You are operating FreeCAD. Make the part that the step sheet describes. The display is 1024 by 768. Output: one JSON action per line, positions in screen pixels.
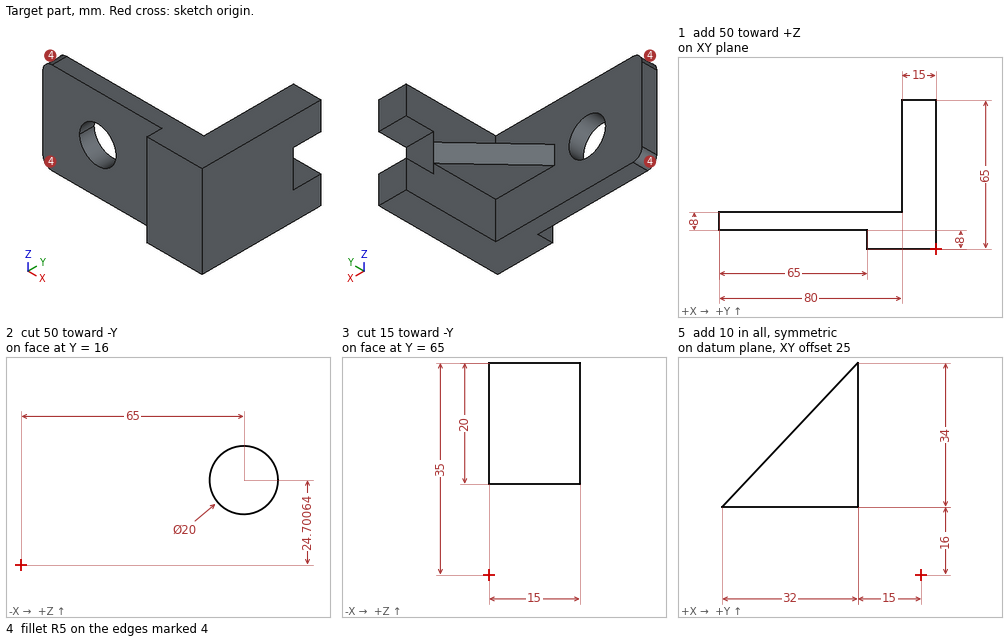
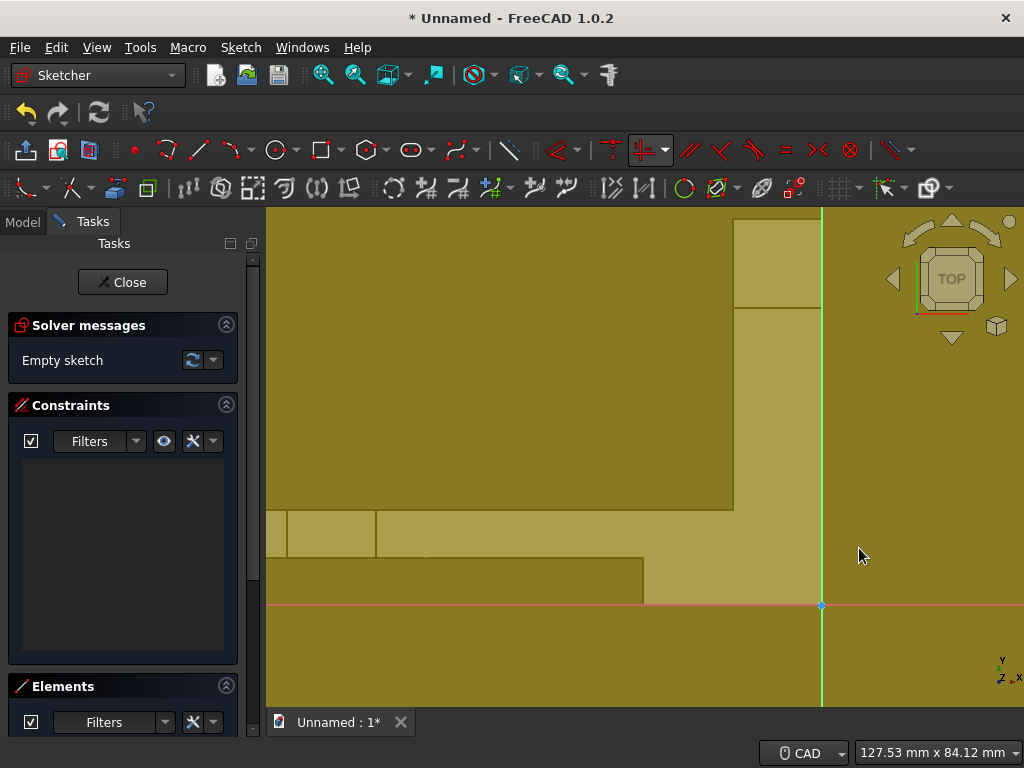
{"action": "left_click", "coordinate": [168, 150]}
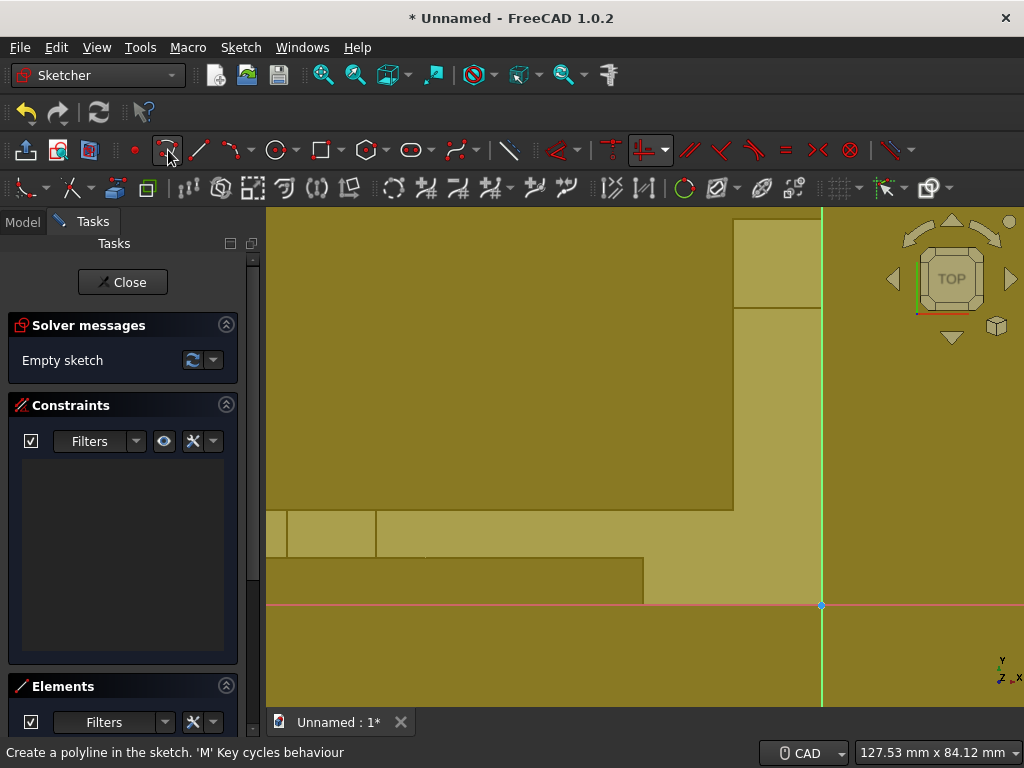
{"action": "left_click", "coordinate": [733, 510]}
{"action": "left_click", "coordinate": [542, 510]}
{"action": "left_click", "coordinate": [733, 308]}
{"action": "left_click", "coordinate": [733, 511]}
{"action": "key", "text": "Escape"}
{"action": "key", "text": "Escape"}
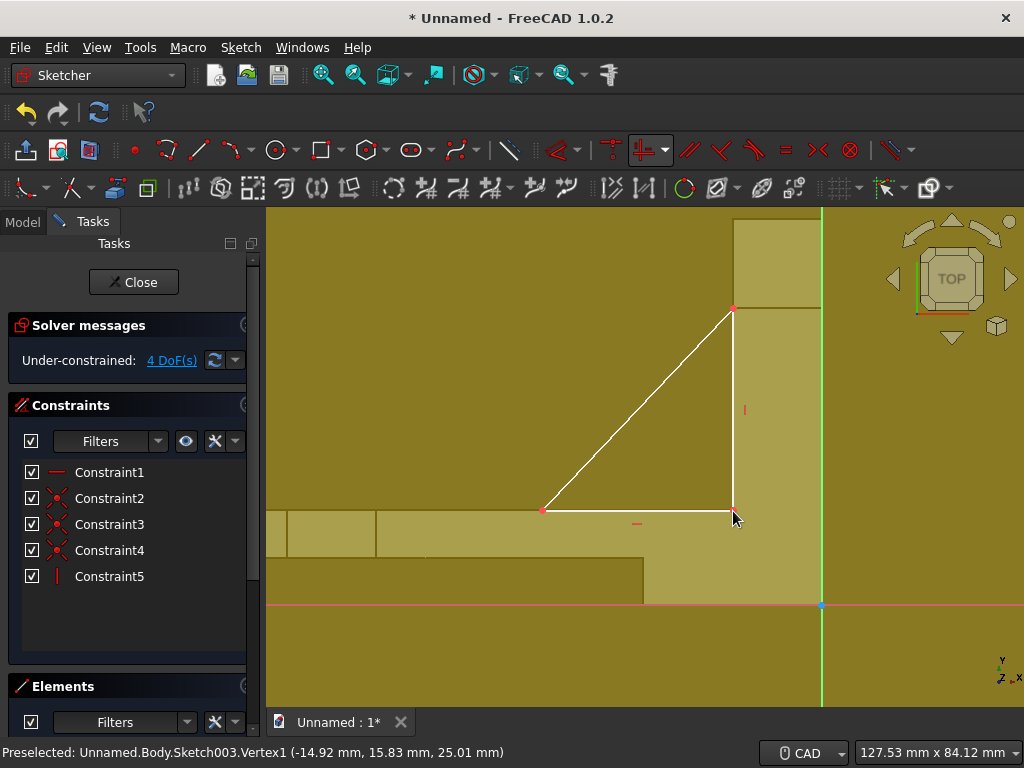
{"action": "key", "text": "d"}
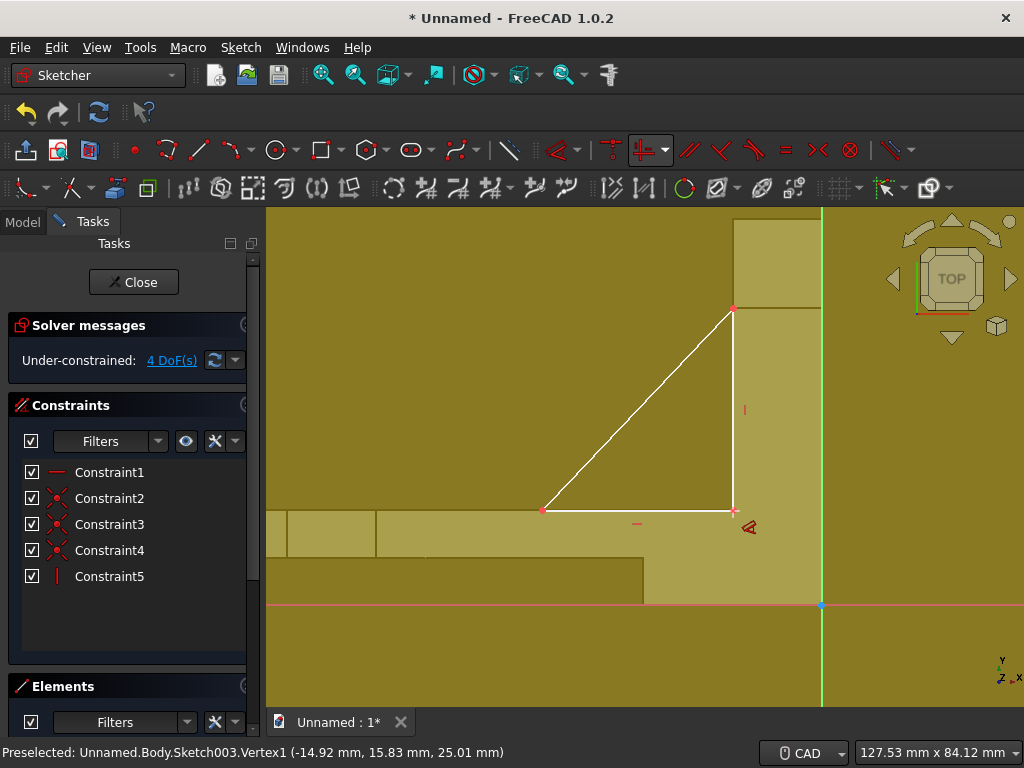
{"action": "left_click", "coordinate": [676, 511]}
{"action": "left_click", "coordinate": [637, 545]}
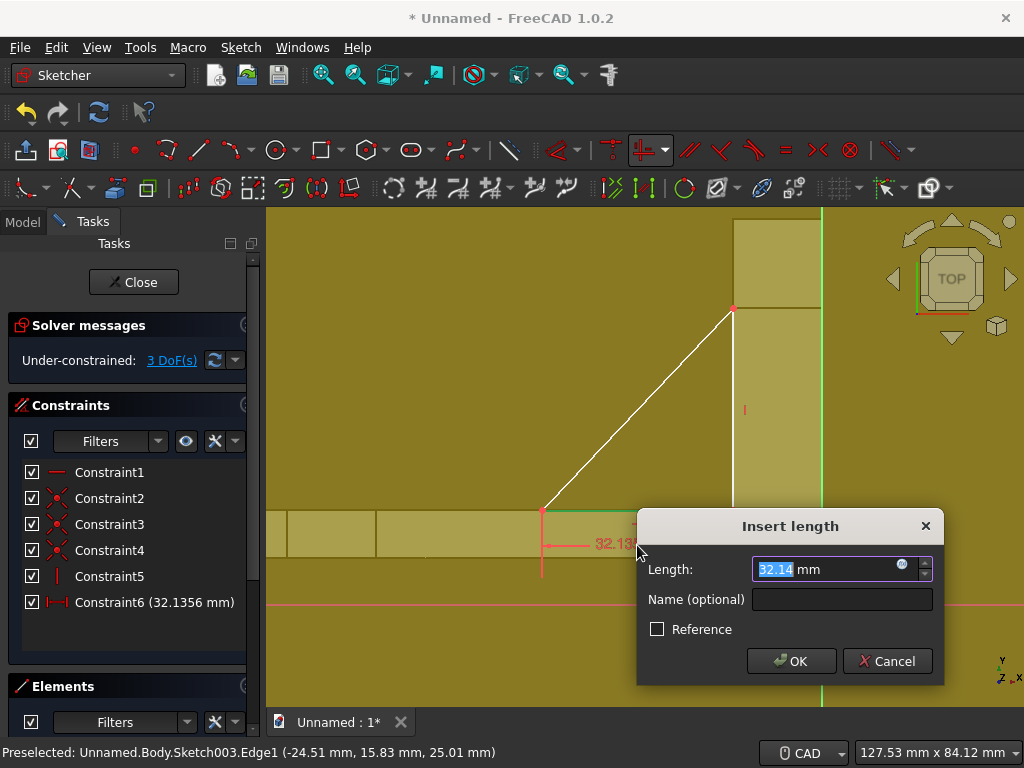
{"action": "type", "text": "32"}
{"action": "key", "text": "Return"}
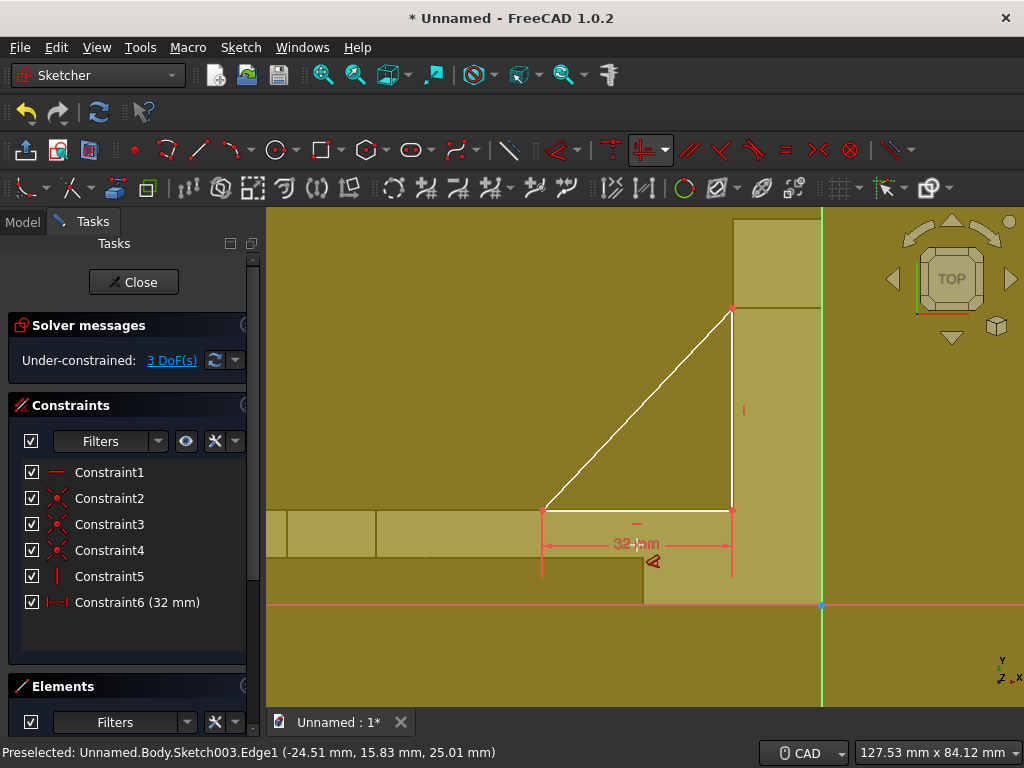
{"action": "left_click", "coordinate": [732, 370]}
{"action": "left_click", "coordinate": [766, 410]}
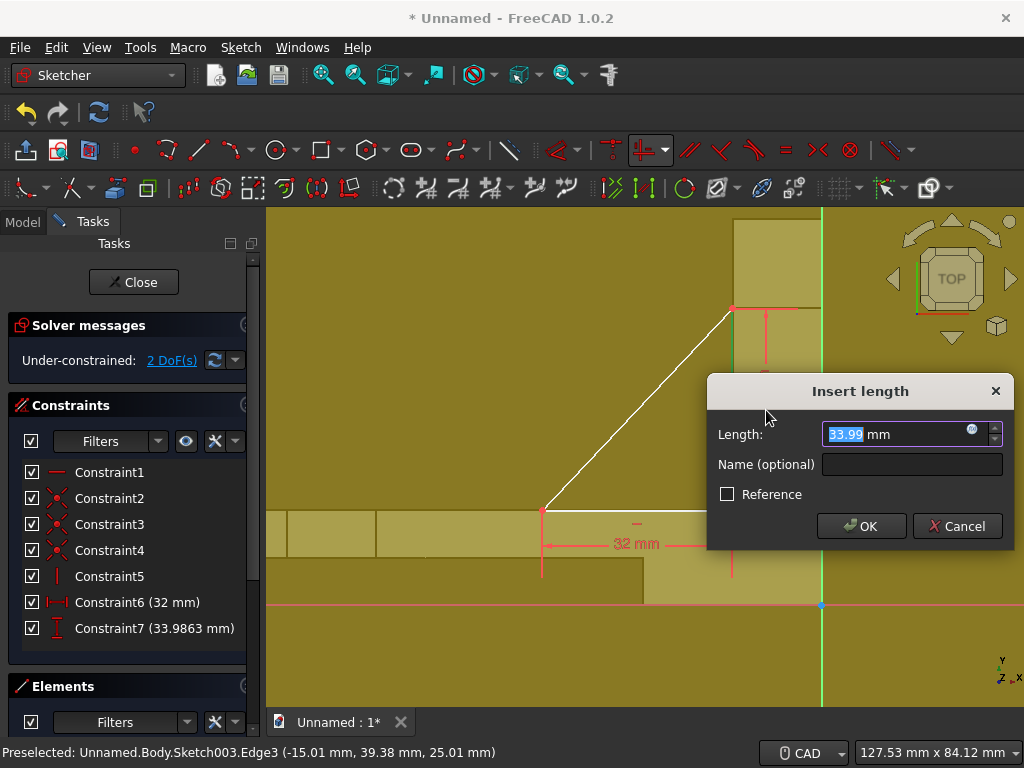
{"action": "type", "text": "34"}
{"action": "key", "text": "Return"}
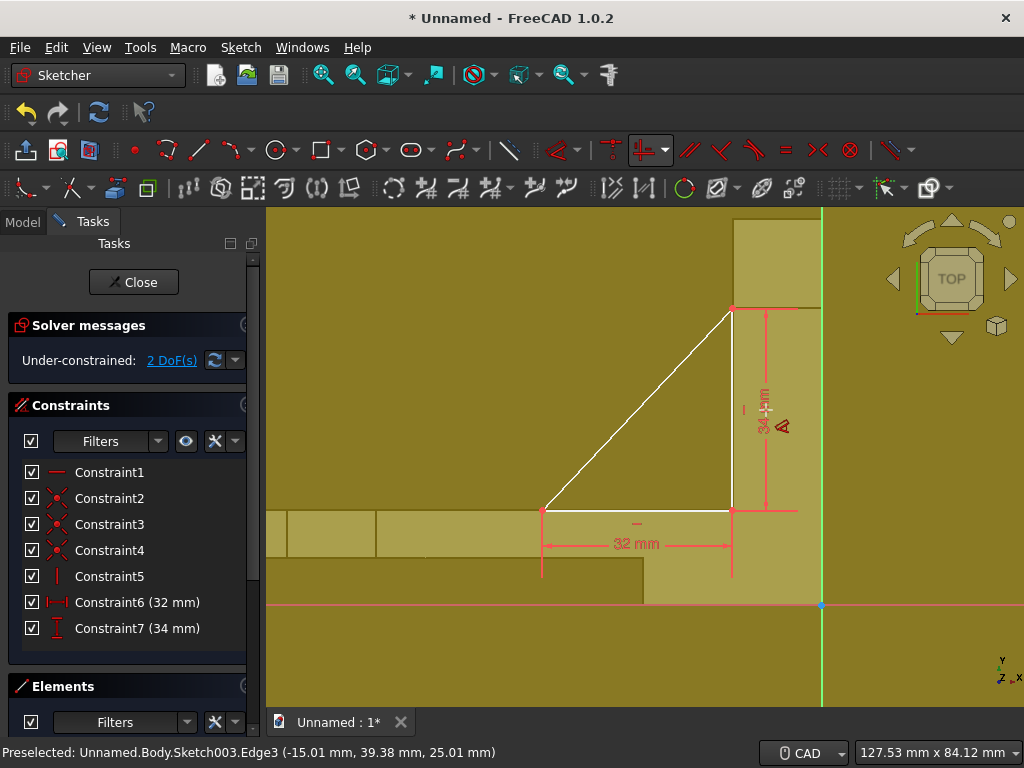
{"action": "left_click", "coordinate": [732, 511]}
{"action": "left_click", "coordinate": [777, 639]}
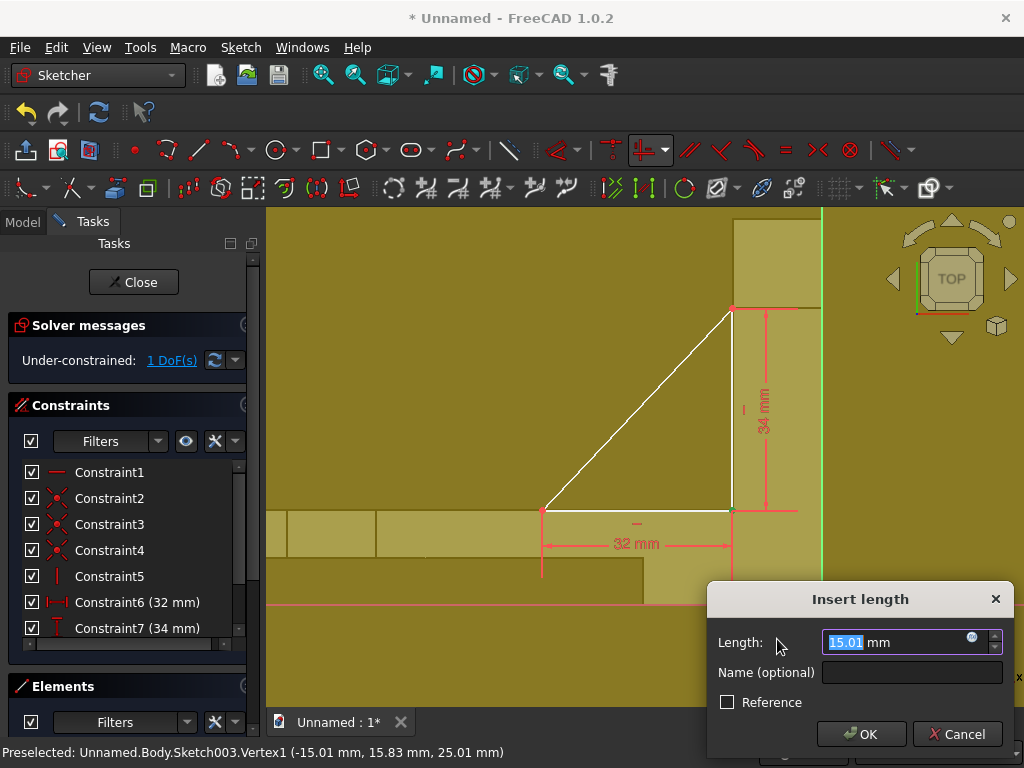
{"action": "type", "text": "15"}
{"action": "key", "text": "Return"}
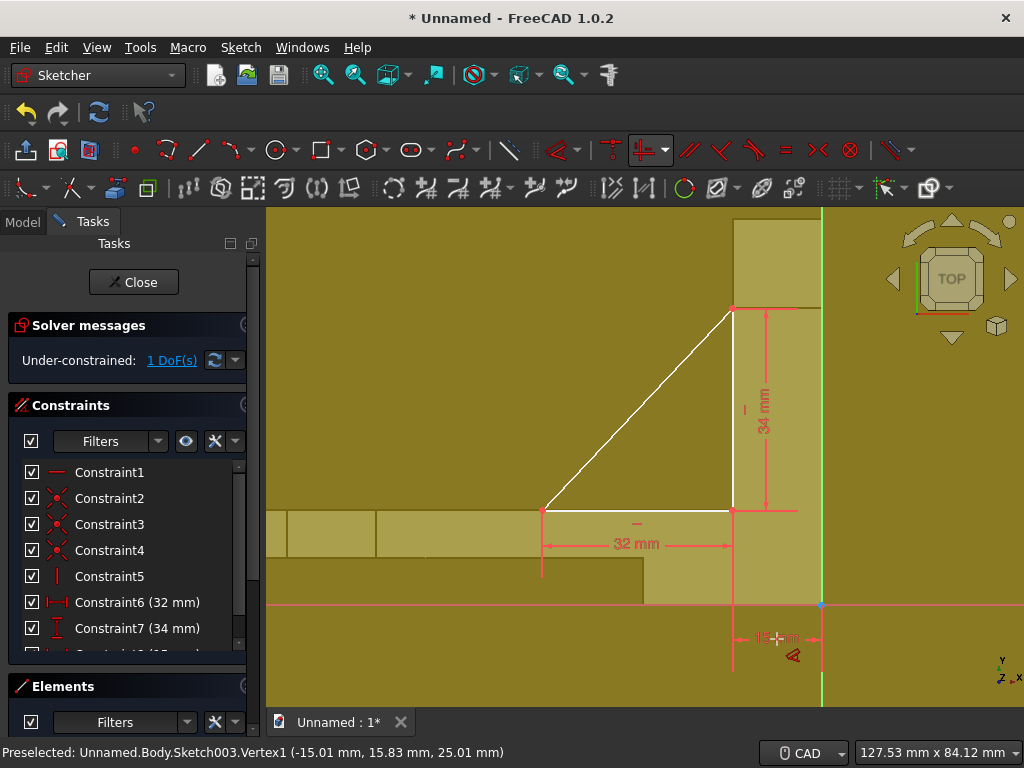
{"action": "left_click", "coordinate": [733, 511]}
{"action": "left_click", "coordinate": [856, 558]}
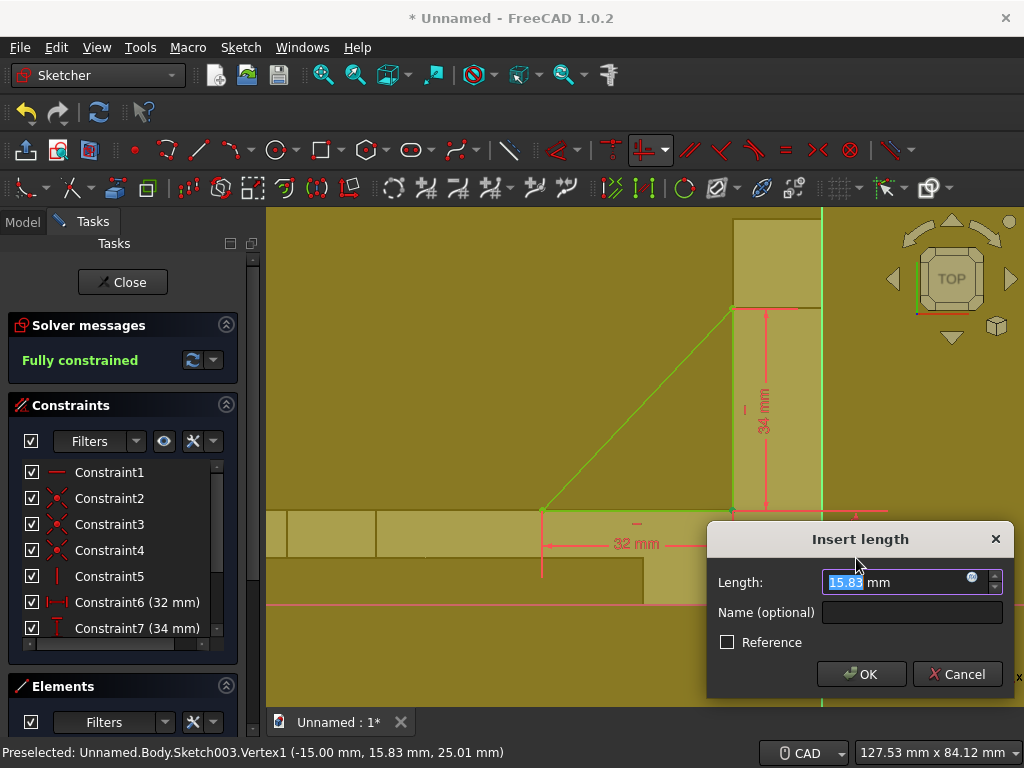
{"action": "type", "text": "16"}
{"action": "key", "text": "Return"}
{"action": "key", "text": "Escape"}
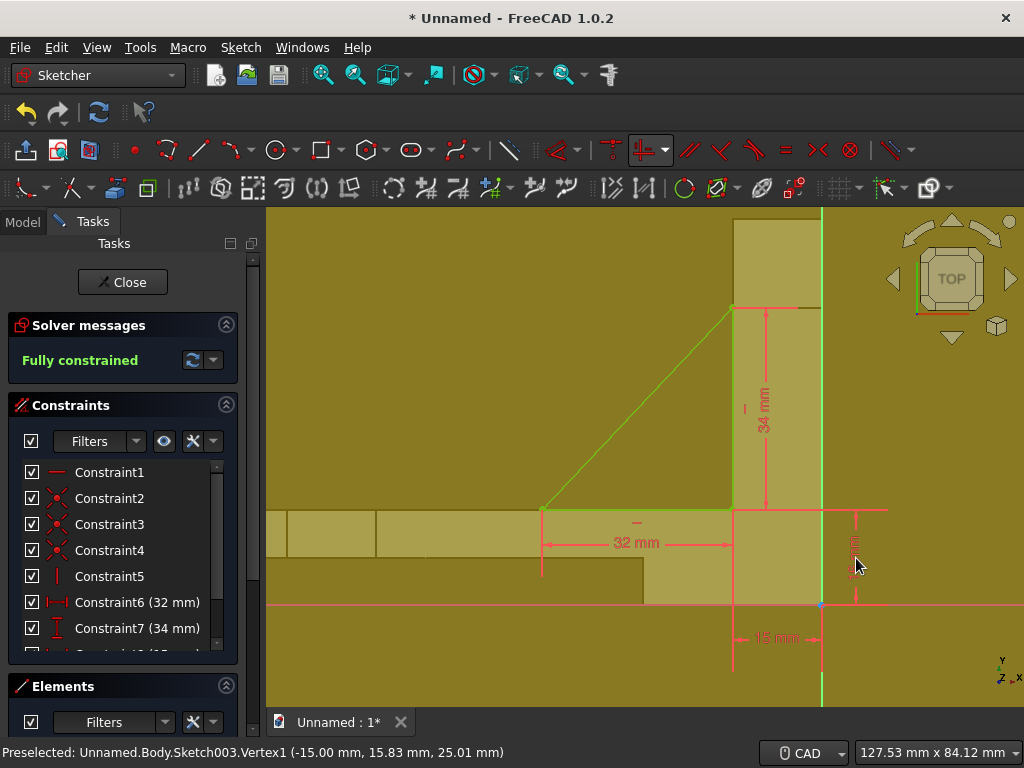
{"action": "left_click", "coordinate": [123, 282]}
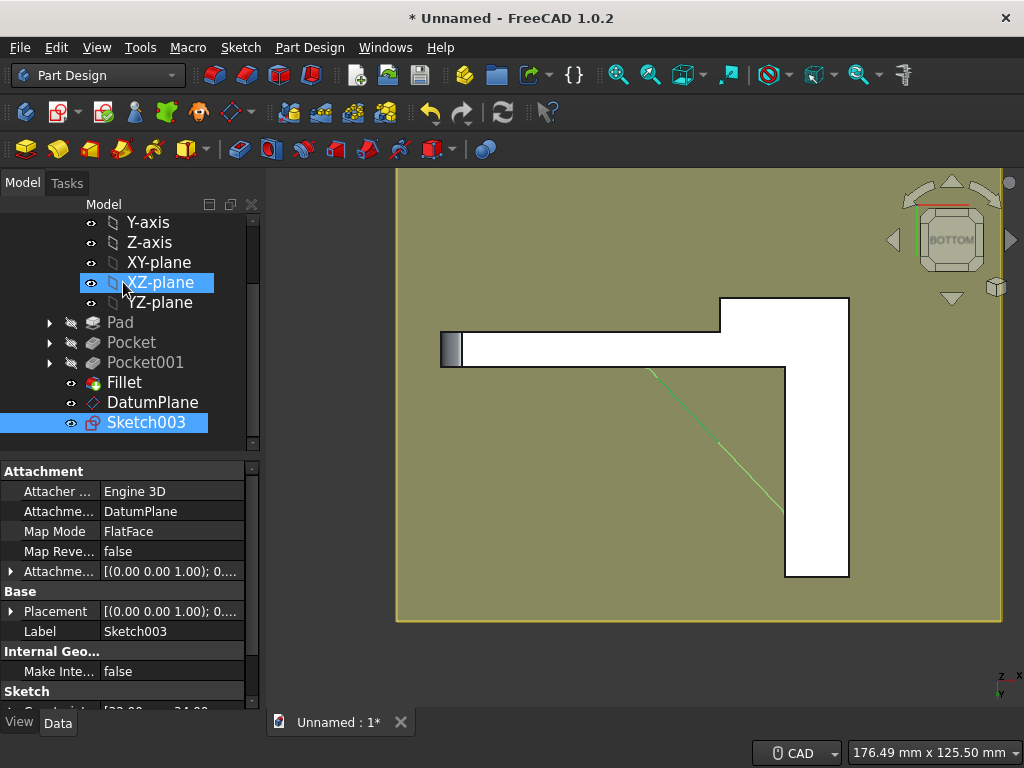
{"action": "left_click", "coordinate": [26, 150]}